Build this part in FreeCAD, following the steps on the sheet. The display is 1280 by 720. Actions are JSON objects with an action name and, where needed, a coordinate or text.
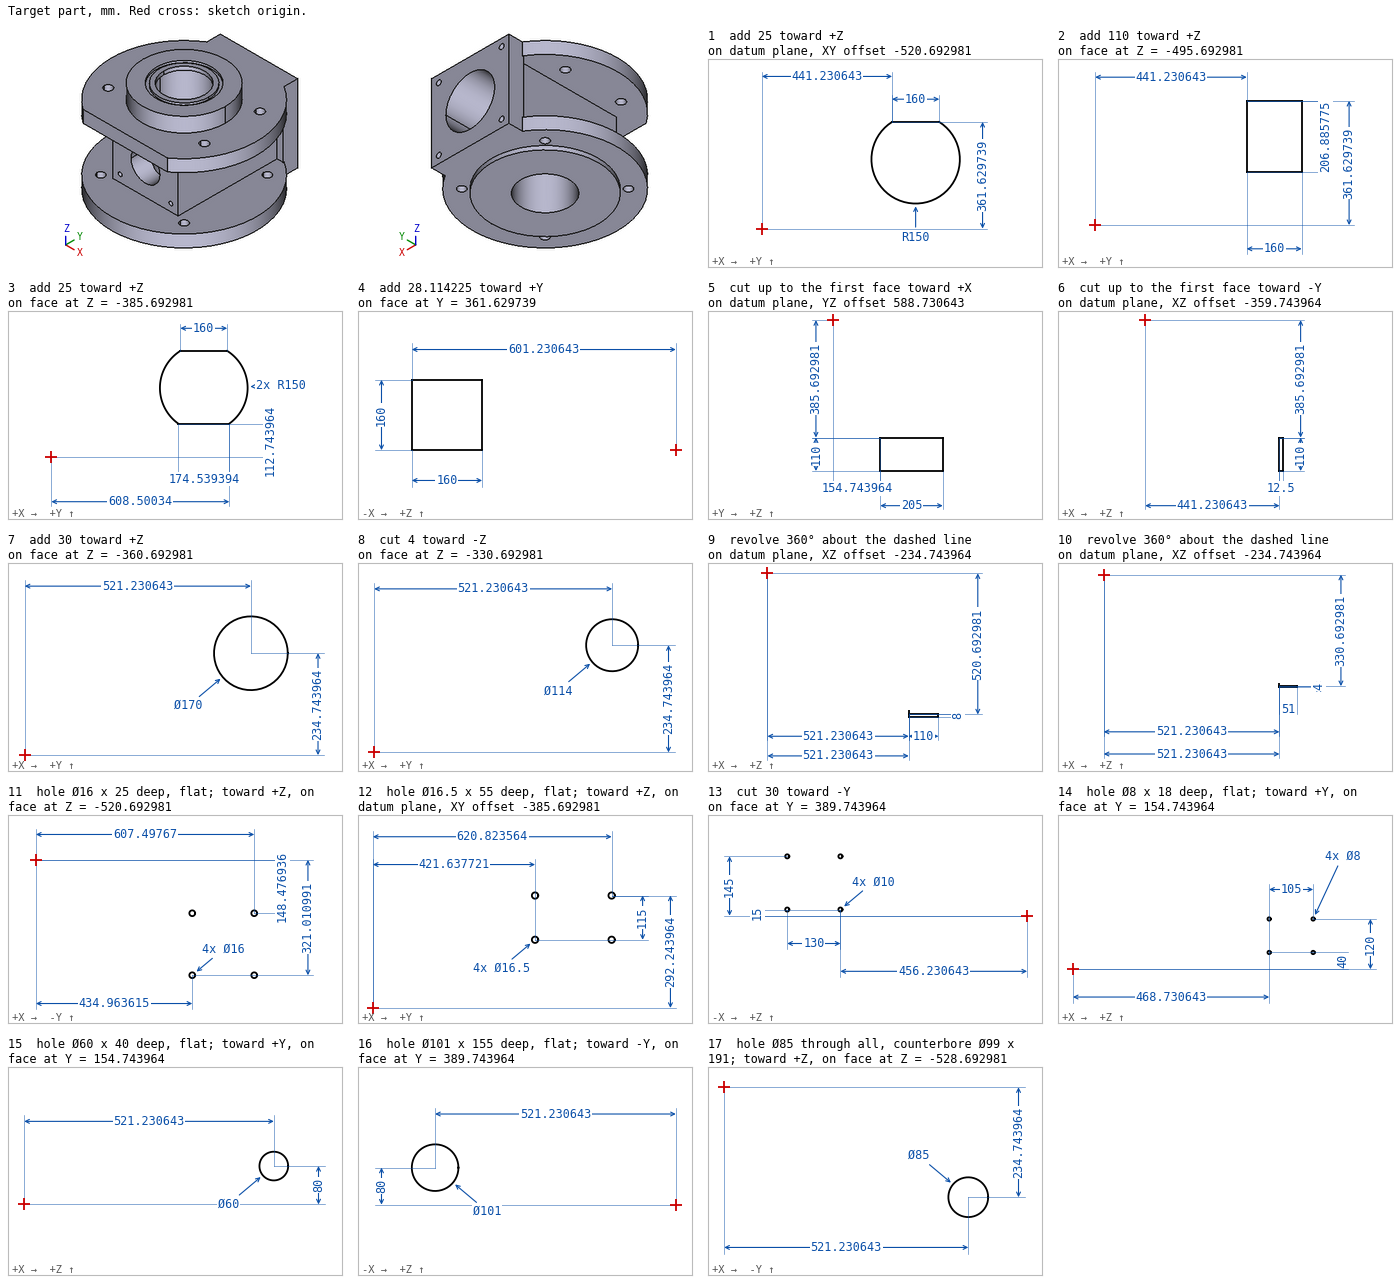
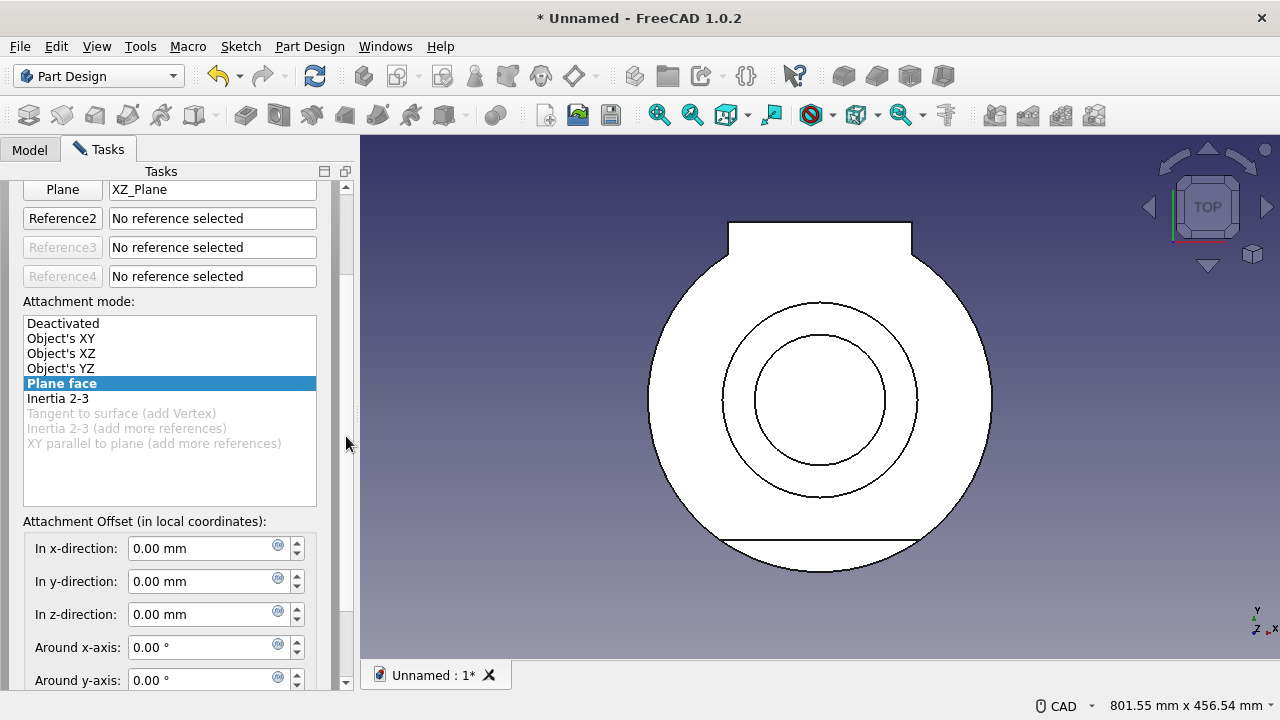
{"action": "triple_click", "coordinate": [210, 614]}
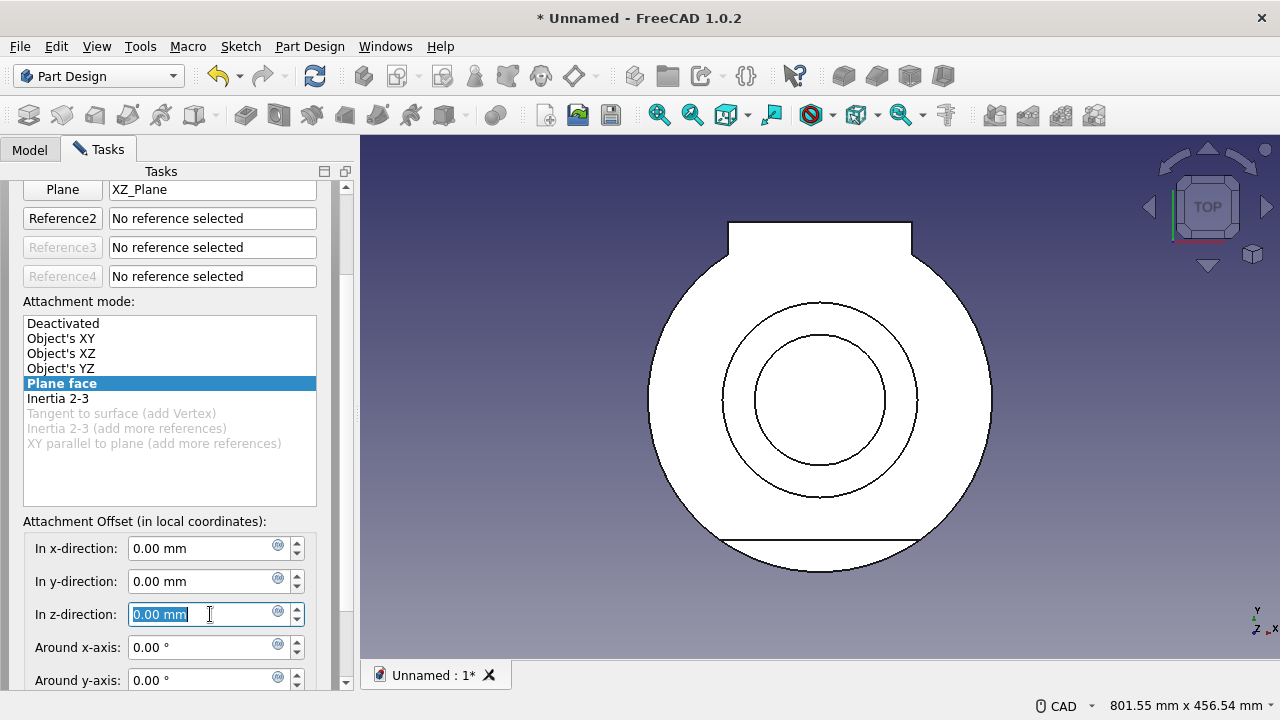
{"action": "type", "text": "-234.743964"}
{"action": "key", "text": "Tab"}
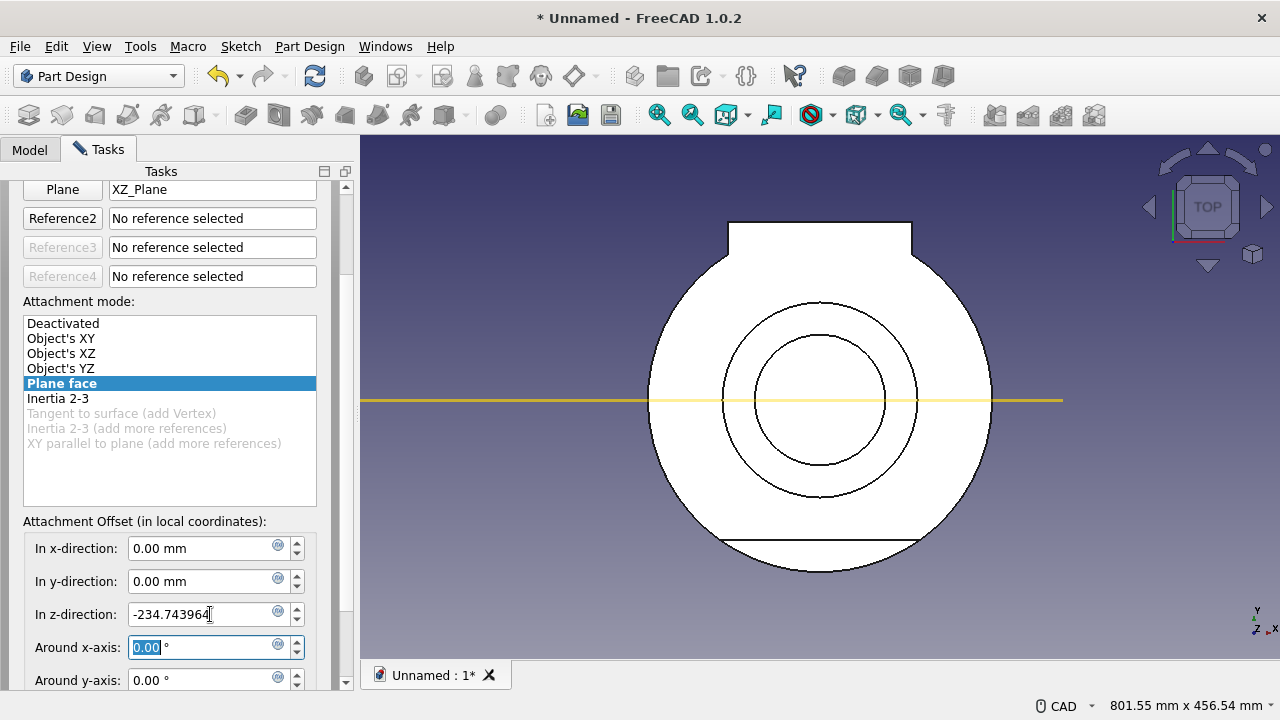
{"action": "scroll", "coordinate": [346, 436], "scroll_direction": "up", "scroll_amount": 3}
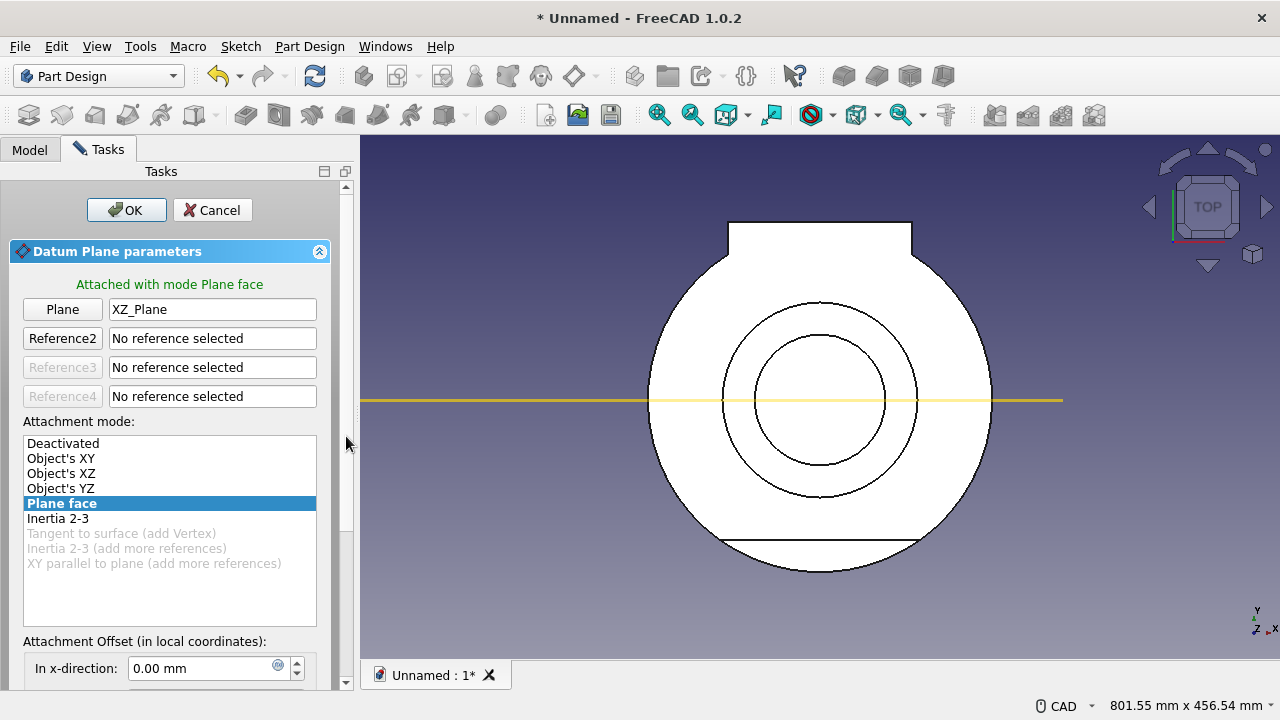
{"action": "left_click", "coordinate": [127, 210]}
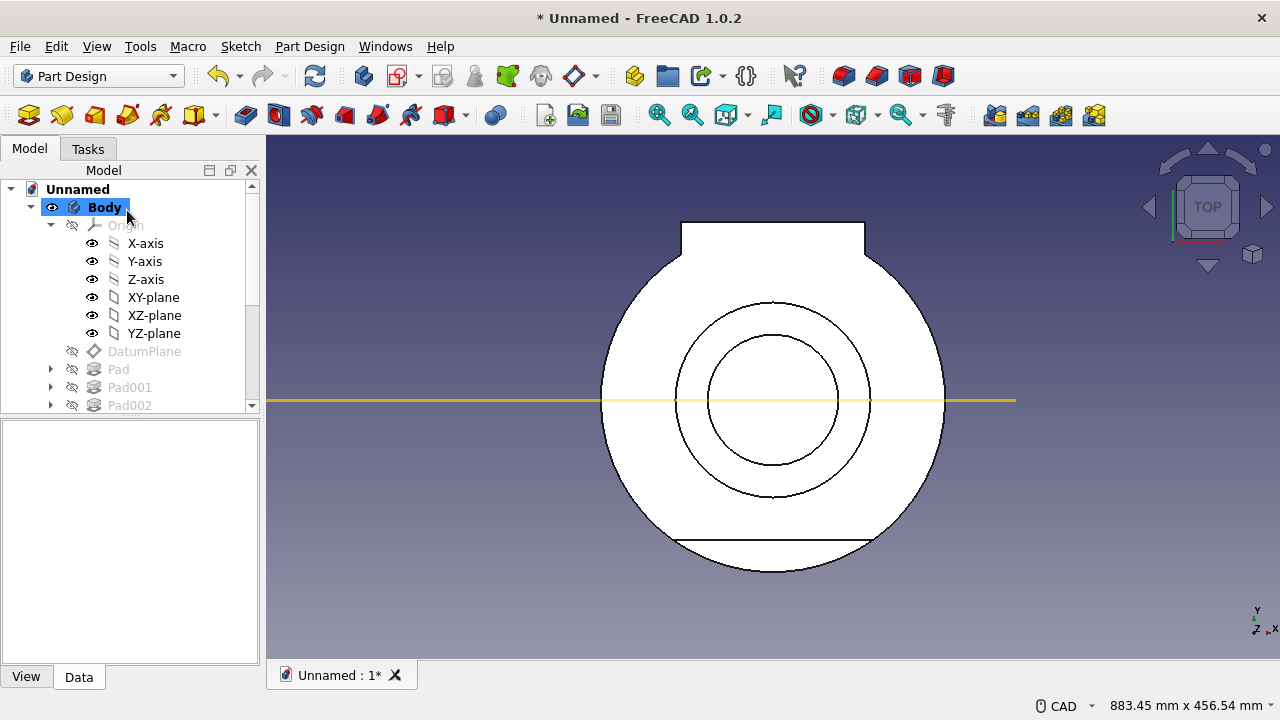
{"action": "scroll", "coordinate": [101, 293], "scroll_direction": "down", "scroll_amount": 3}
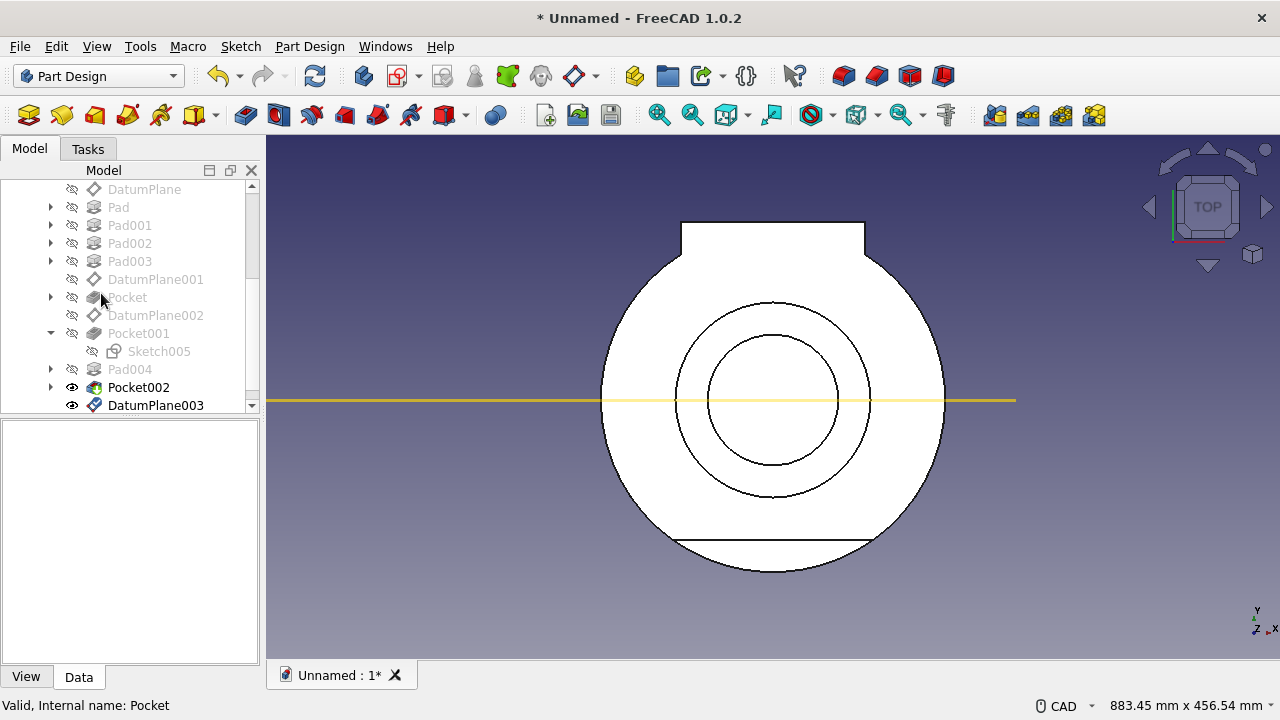
{"action": "left_click", "coordinate": [117, 405]}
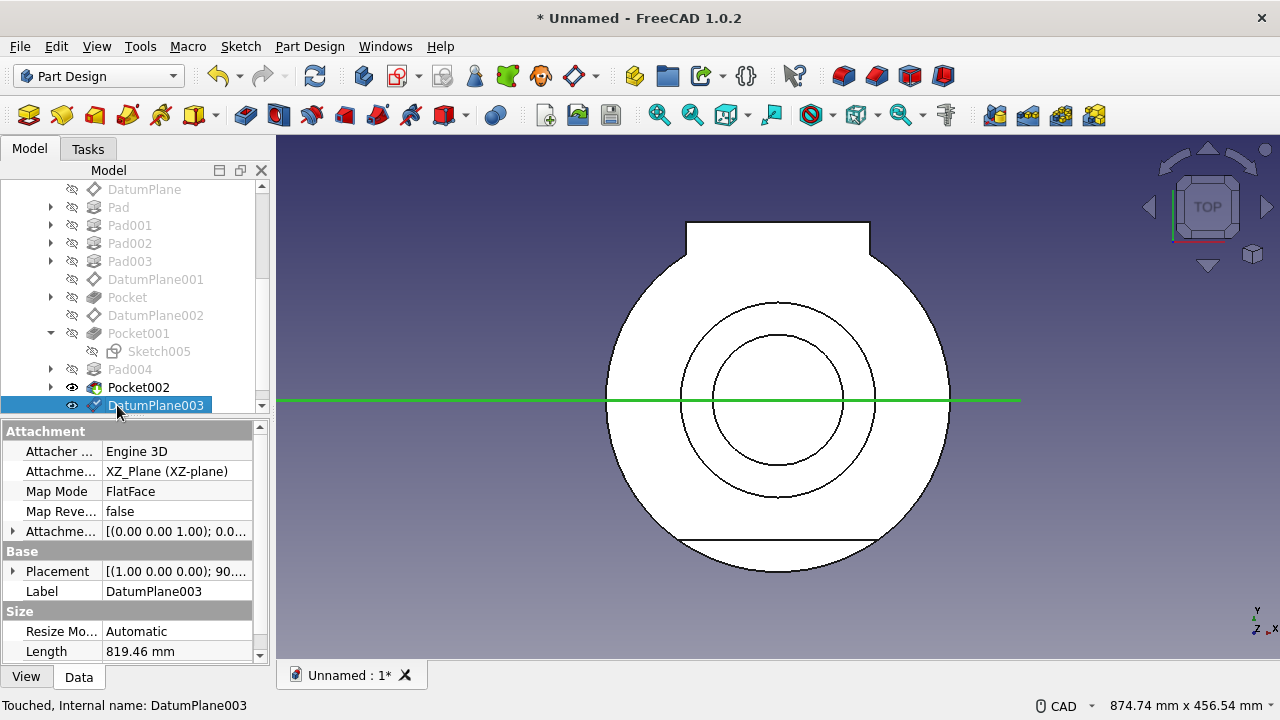
{"action": "left_click", "coordinate": [396, 76]}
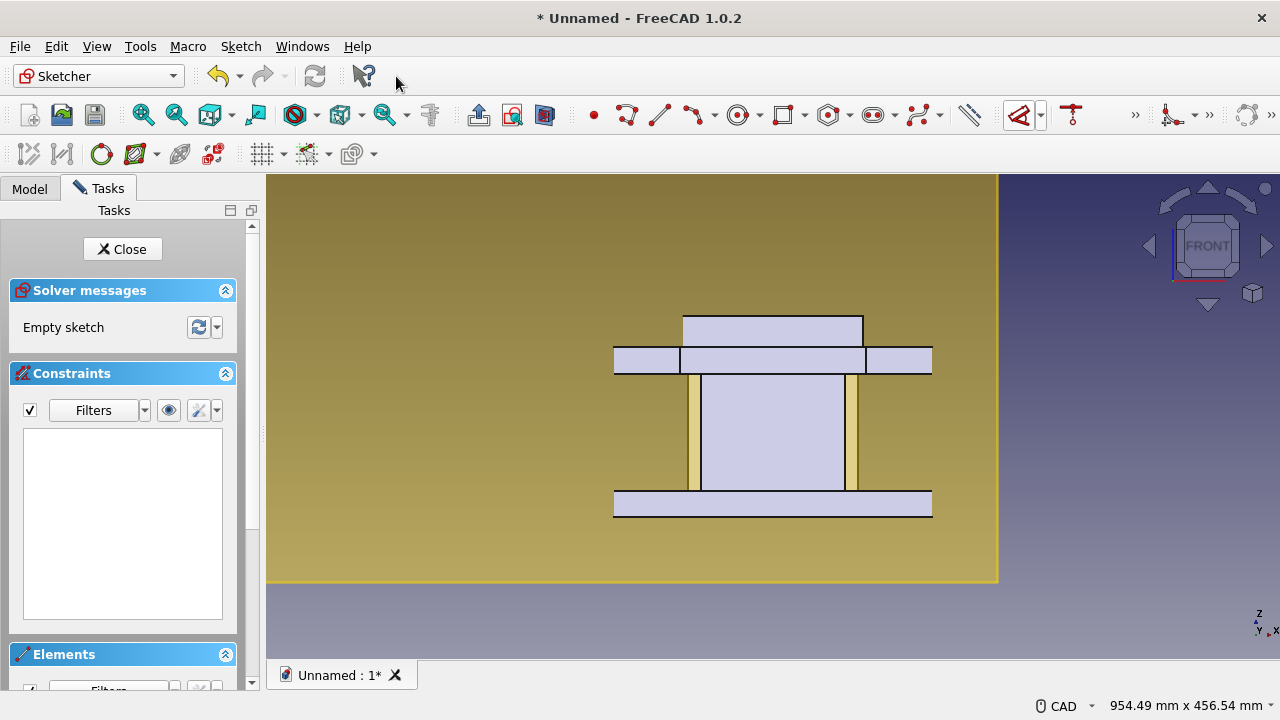
{"action": "left_click", "coordinate": [545, 116]}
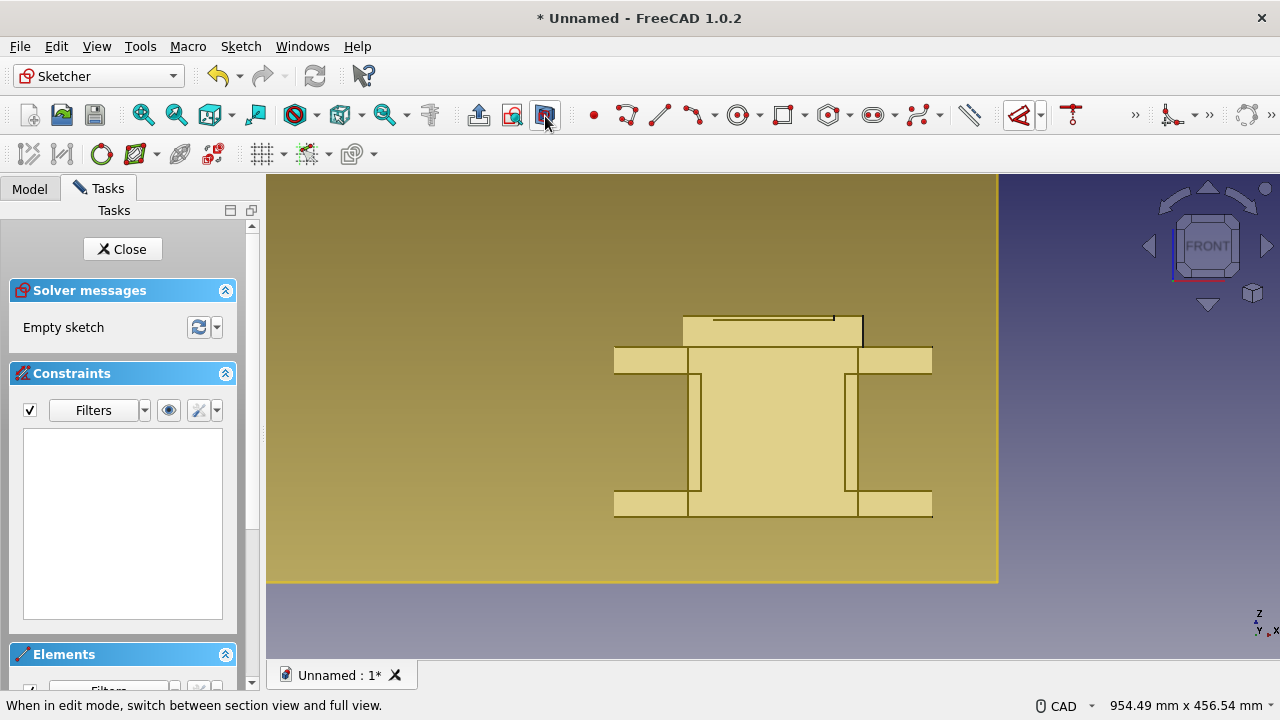
{"action": "scroll", "coordinate": [864, 537], "scroll_direction": "up", "scroll_amount": 8}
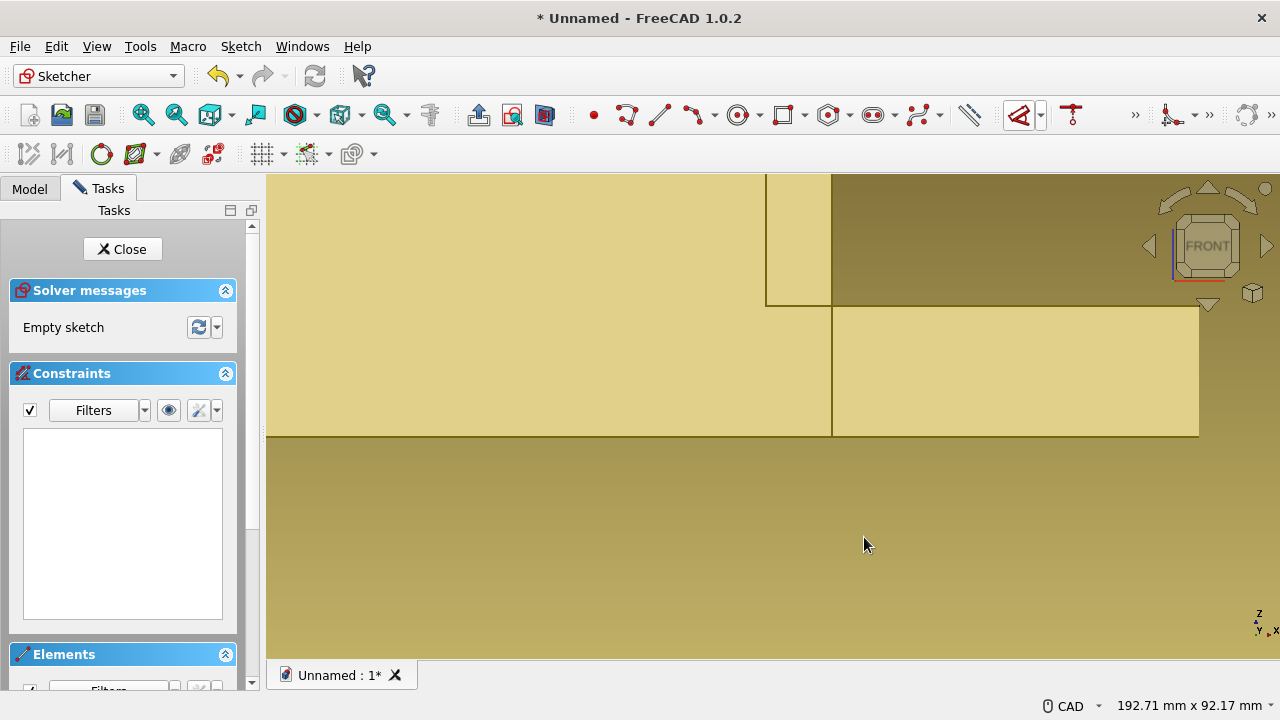
{"action": "left_click", "coordinate": [782, 116]}